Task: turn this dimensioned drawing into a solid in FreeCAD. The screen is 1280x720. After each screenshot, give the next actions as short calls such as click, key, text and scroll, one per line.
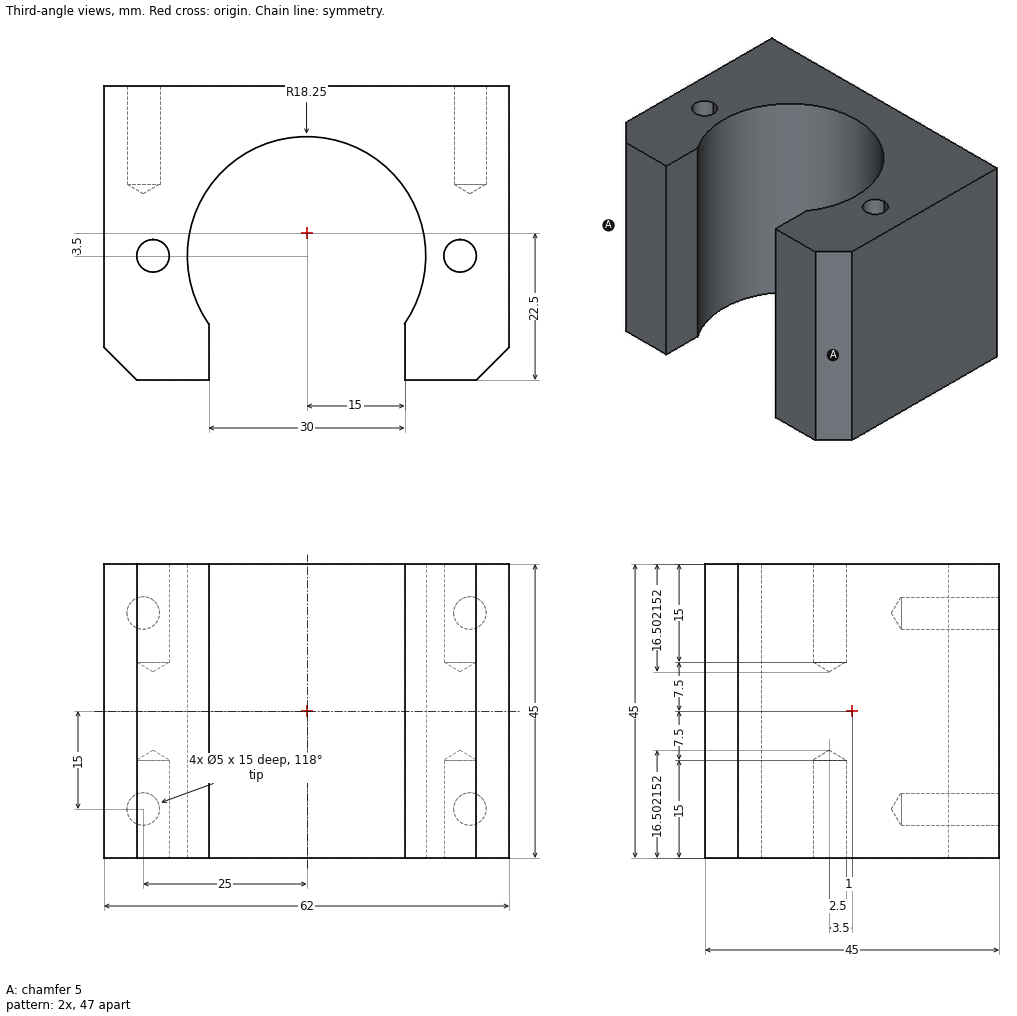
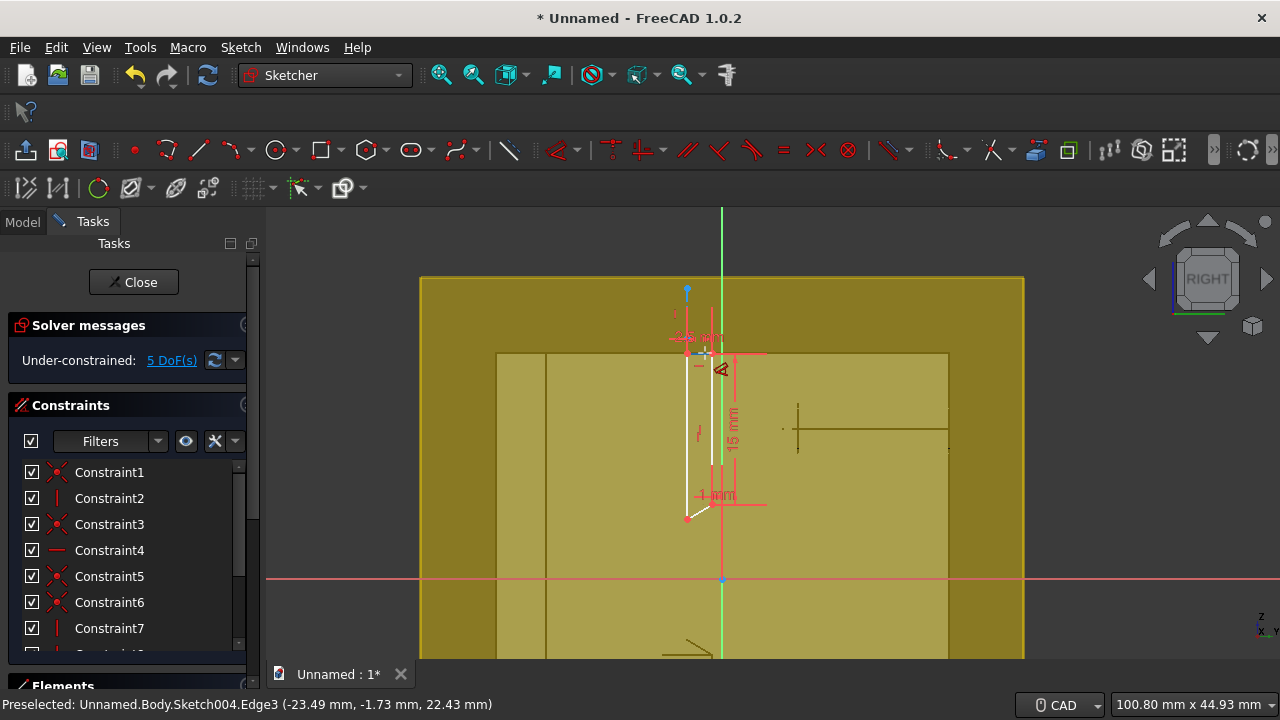
click(712, 505)
click(756, 542)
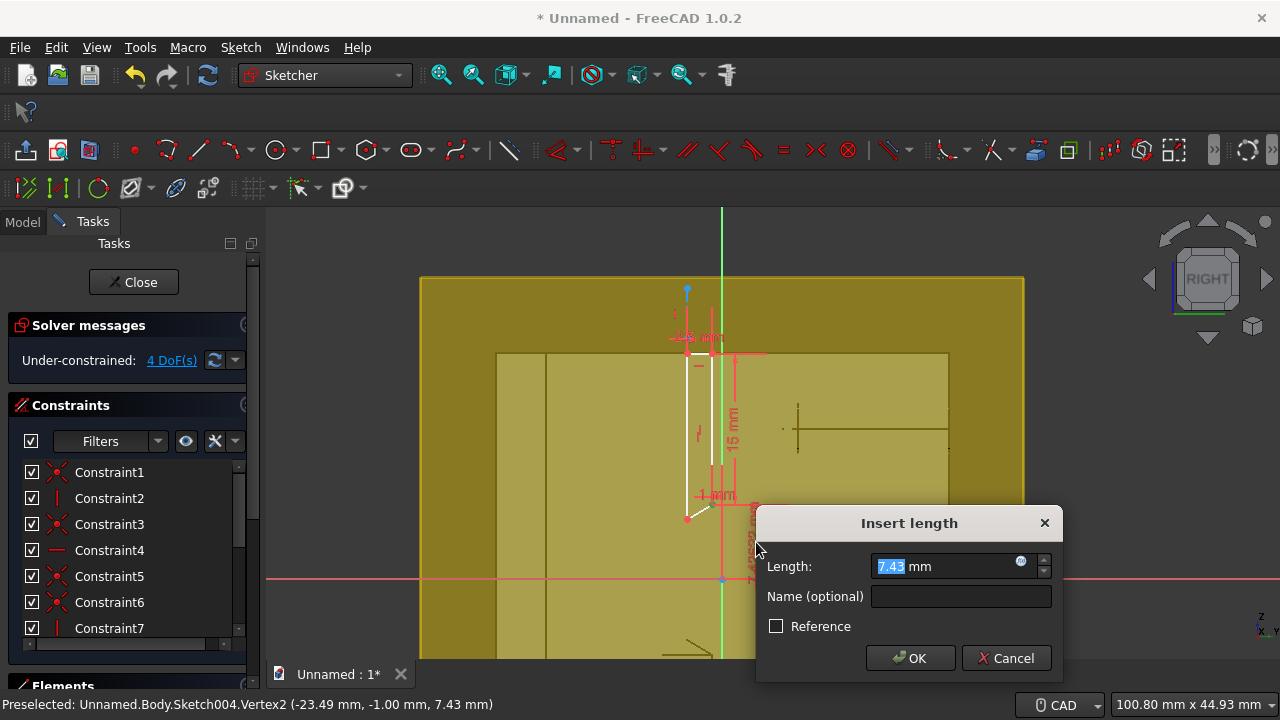
text(7.5)
key(Return)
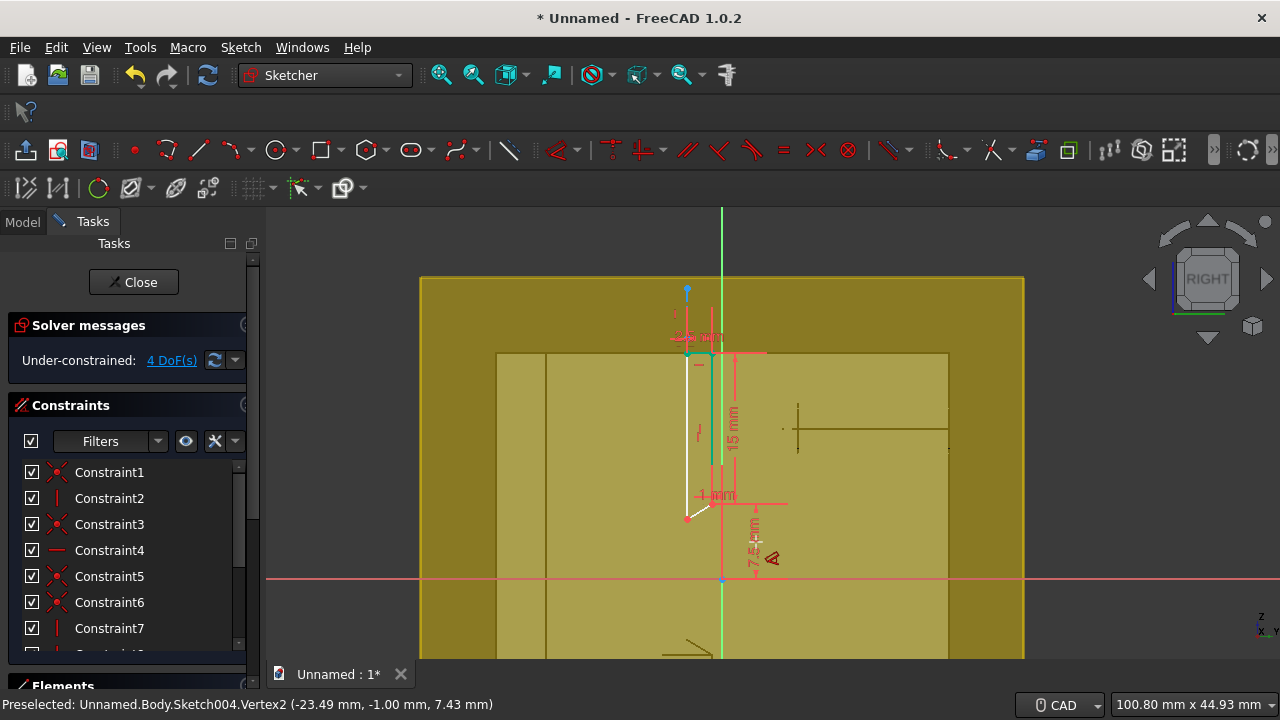
click(687, 338)
click(705, 613)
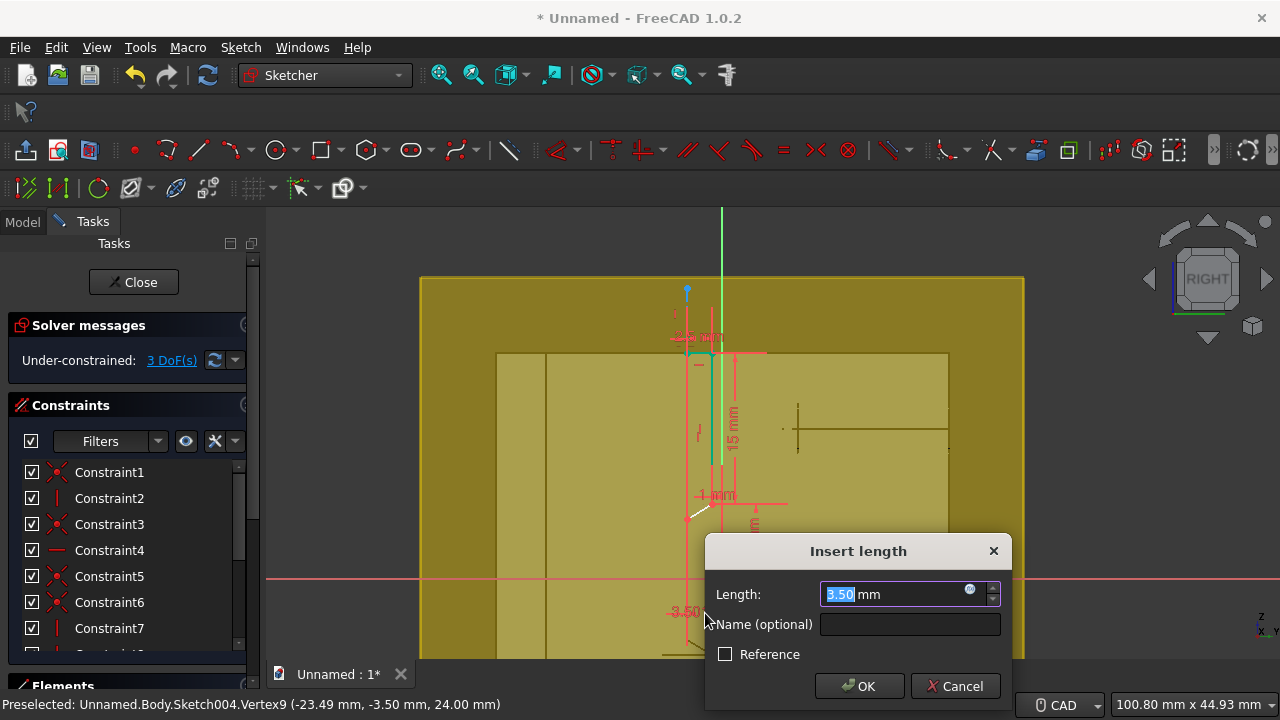
text(3.5)
key(Return)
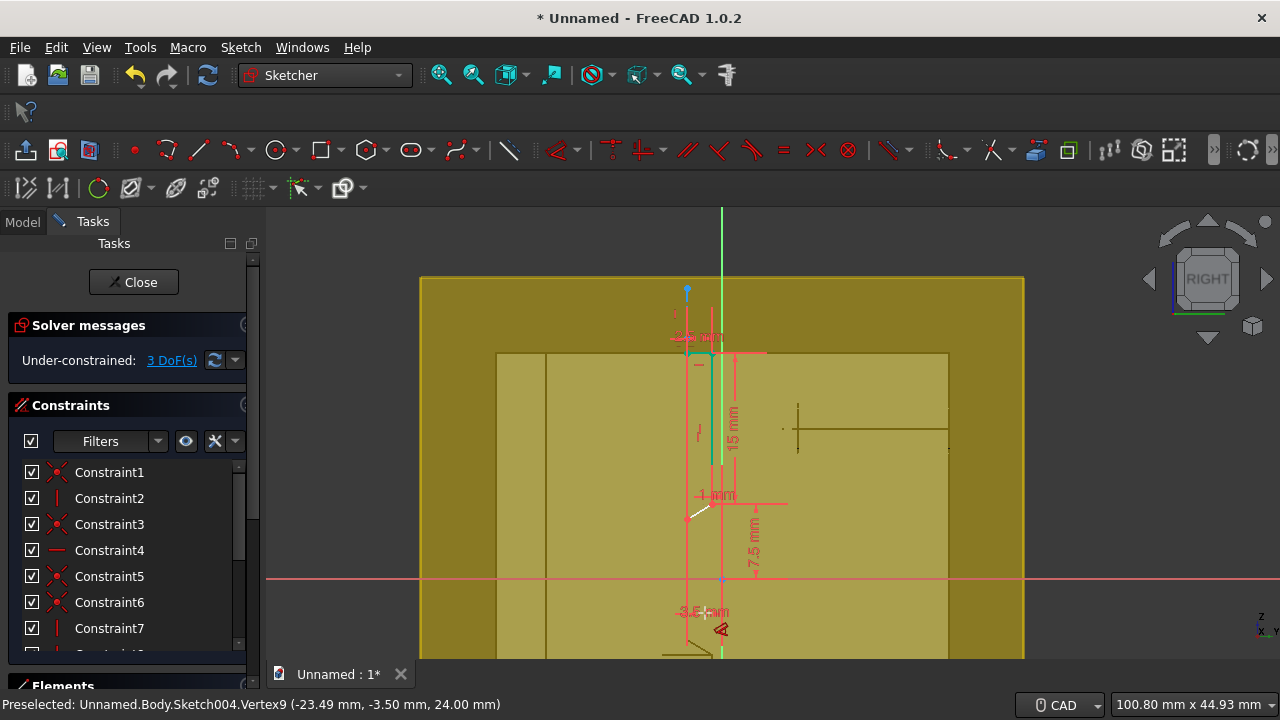
click(687, 403)
click(653, 437)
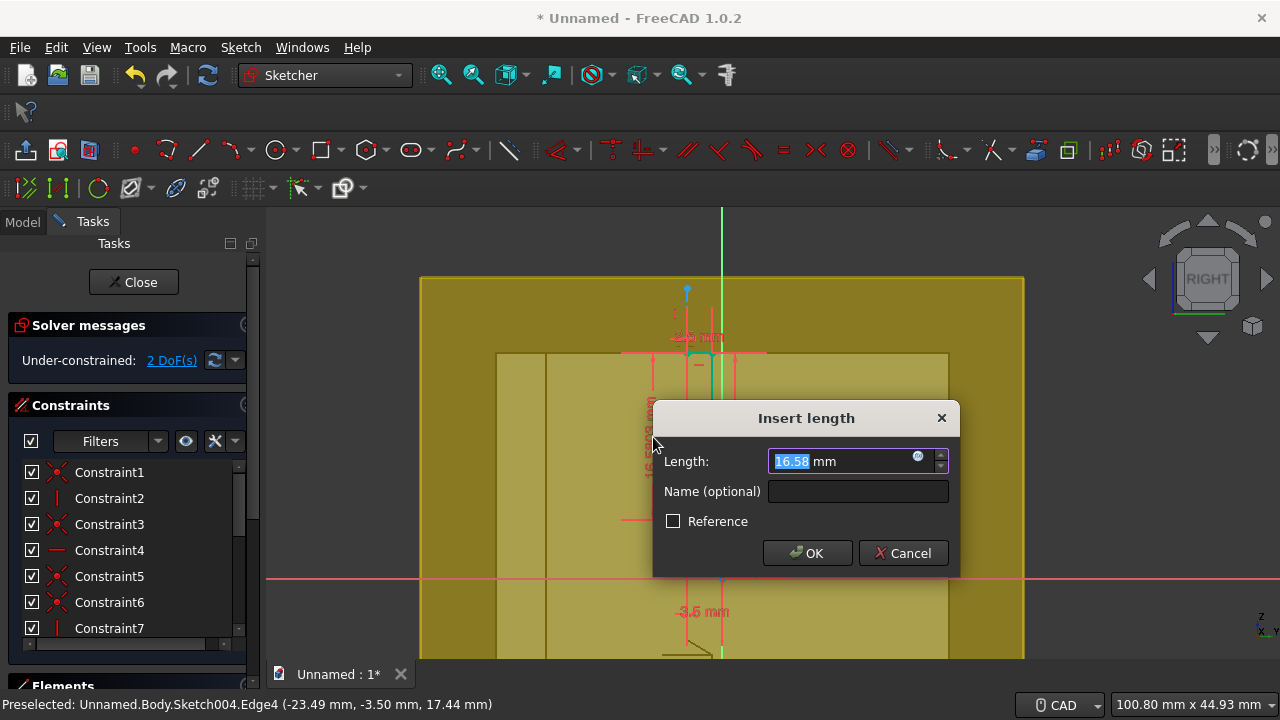
text(16.502152)
key(Return)
key(Escape)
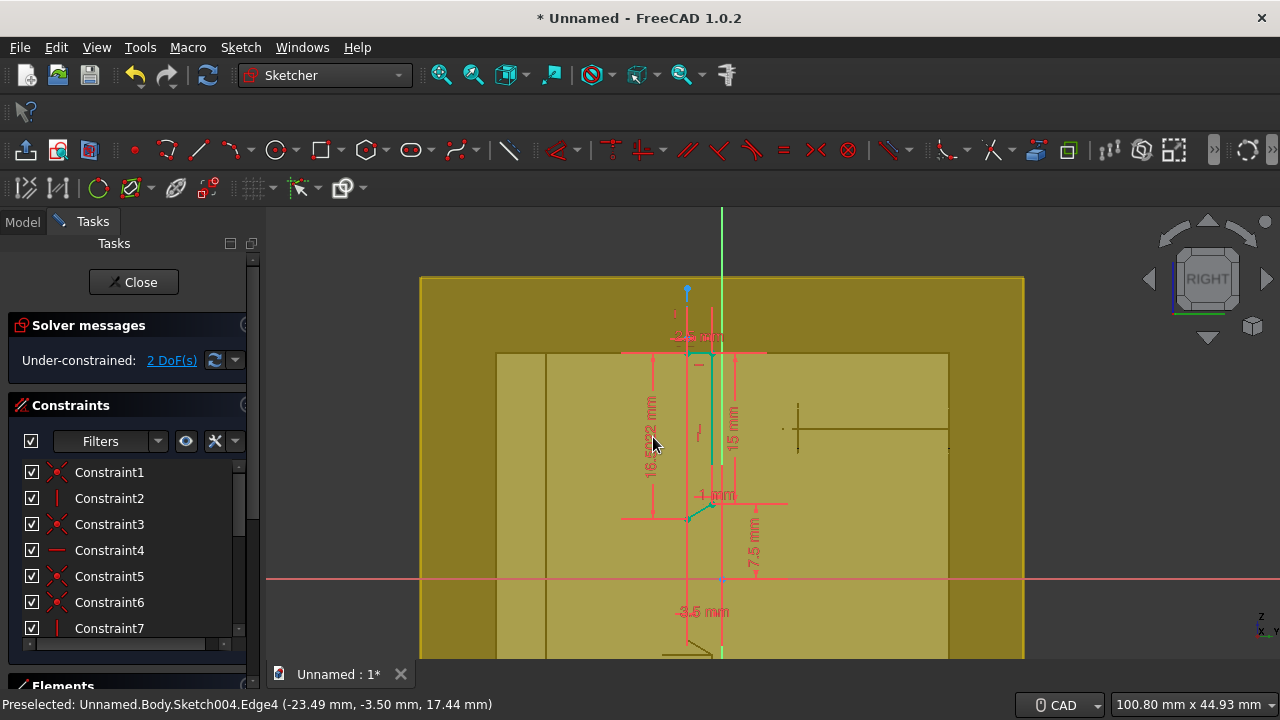
click(134, 282)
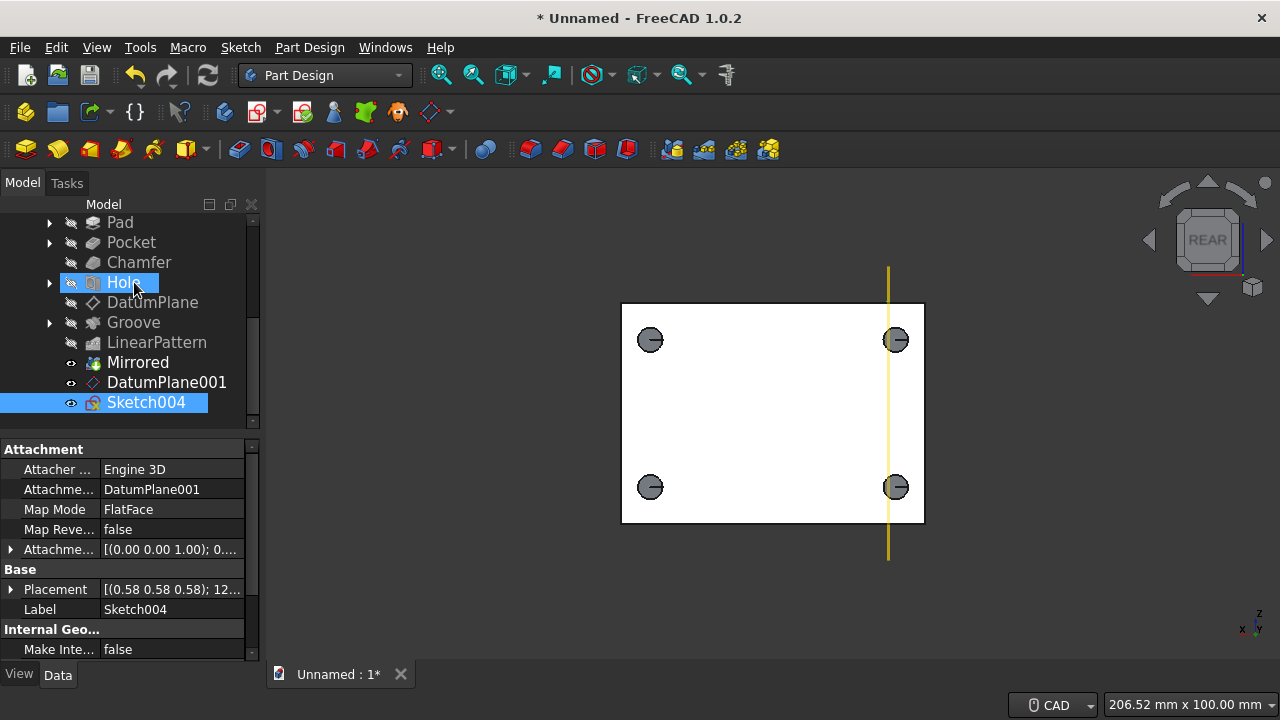
click(304, 150)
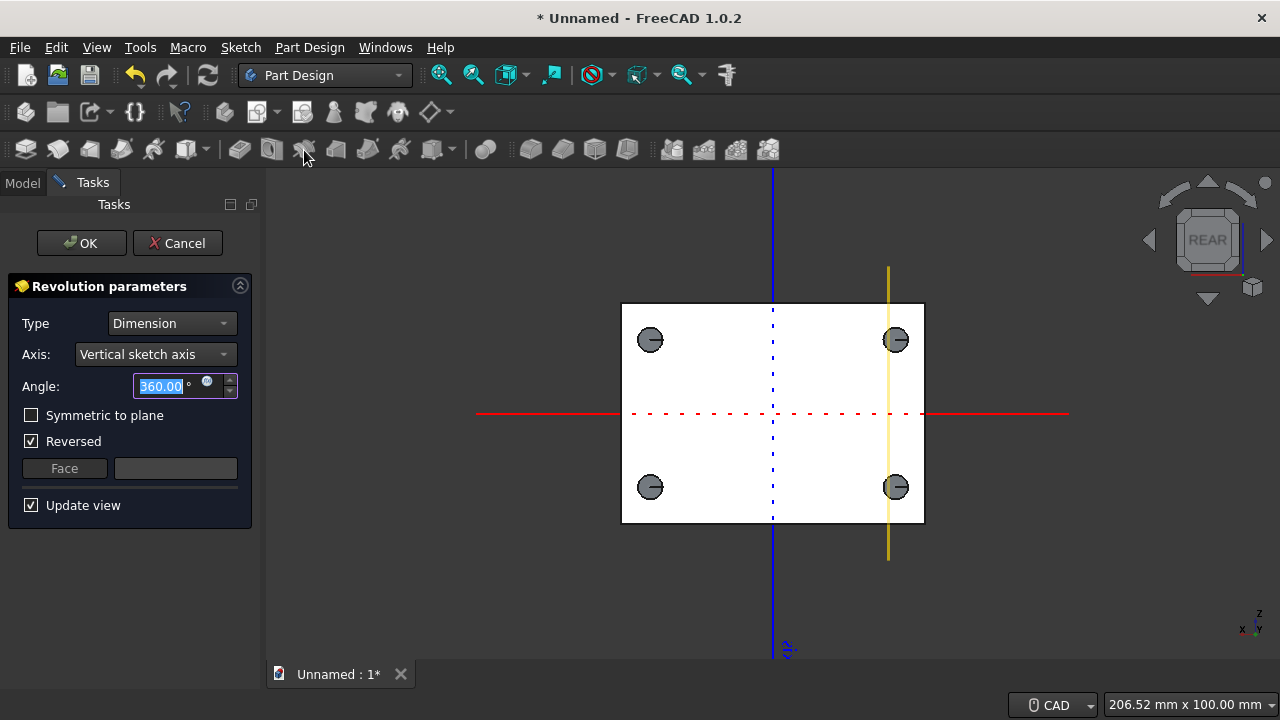
click(156, 354)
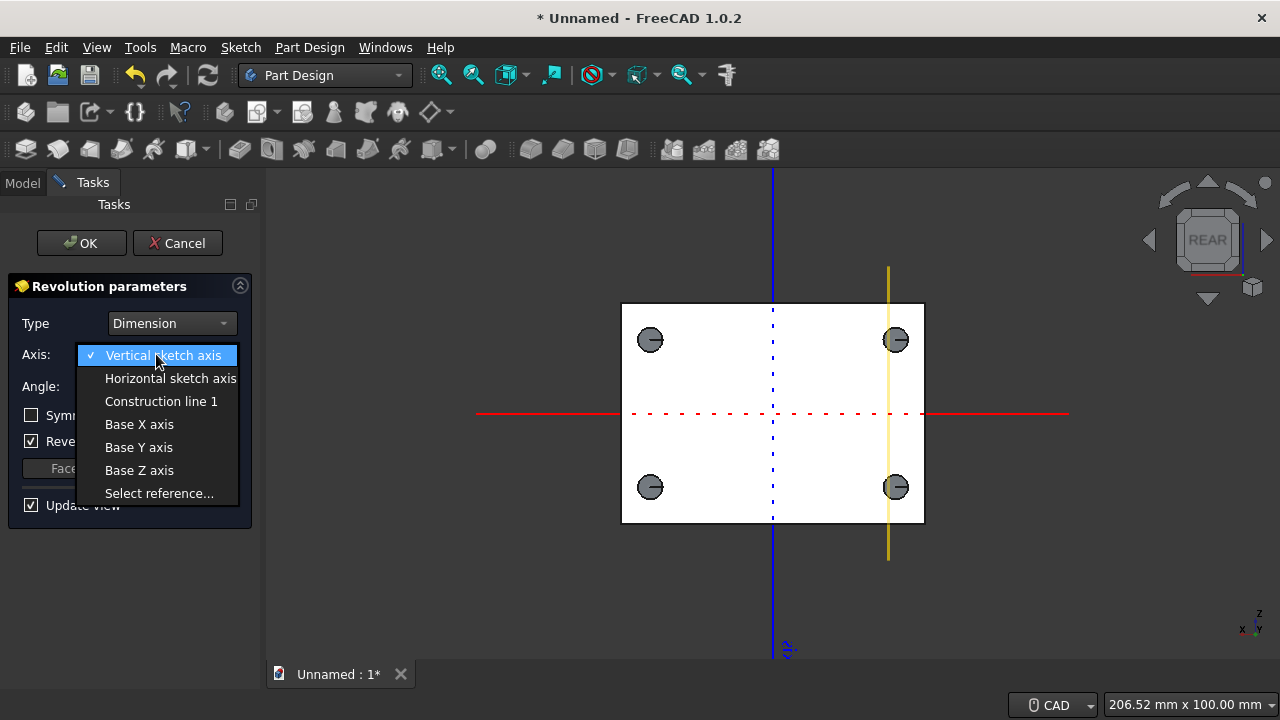
click(156, 402)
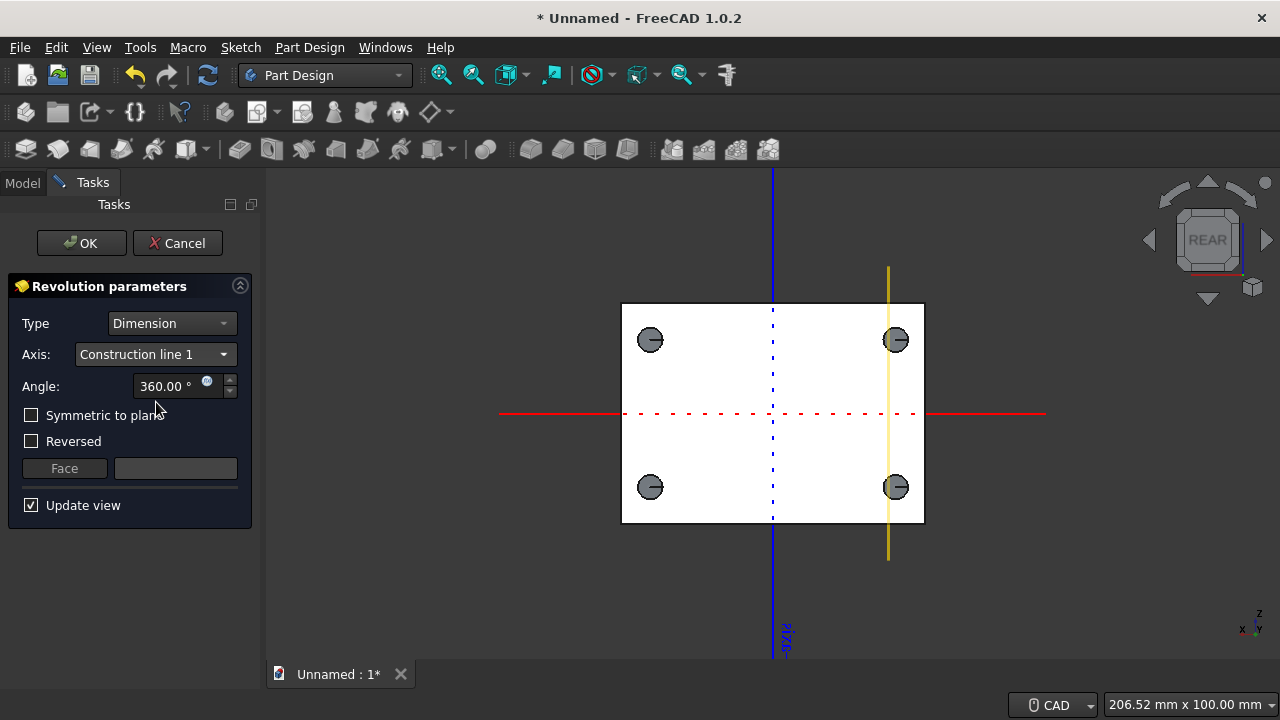
click(82, 243)